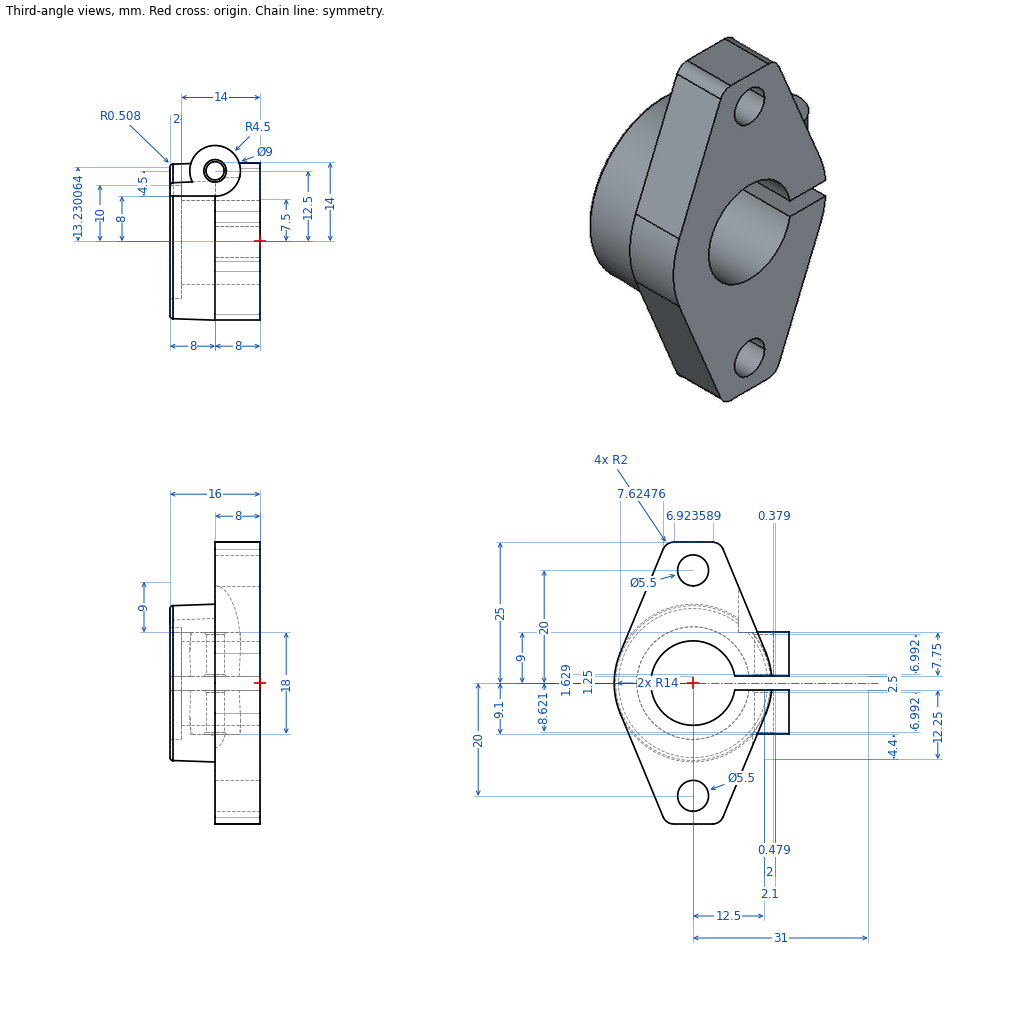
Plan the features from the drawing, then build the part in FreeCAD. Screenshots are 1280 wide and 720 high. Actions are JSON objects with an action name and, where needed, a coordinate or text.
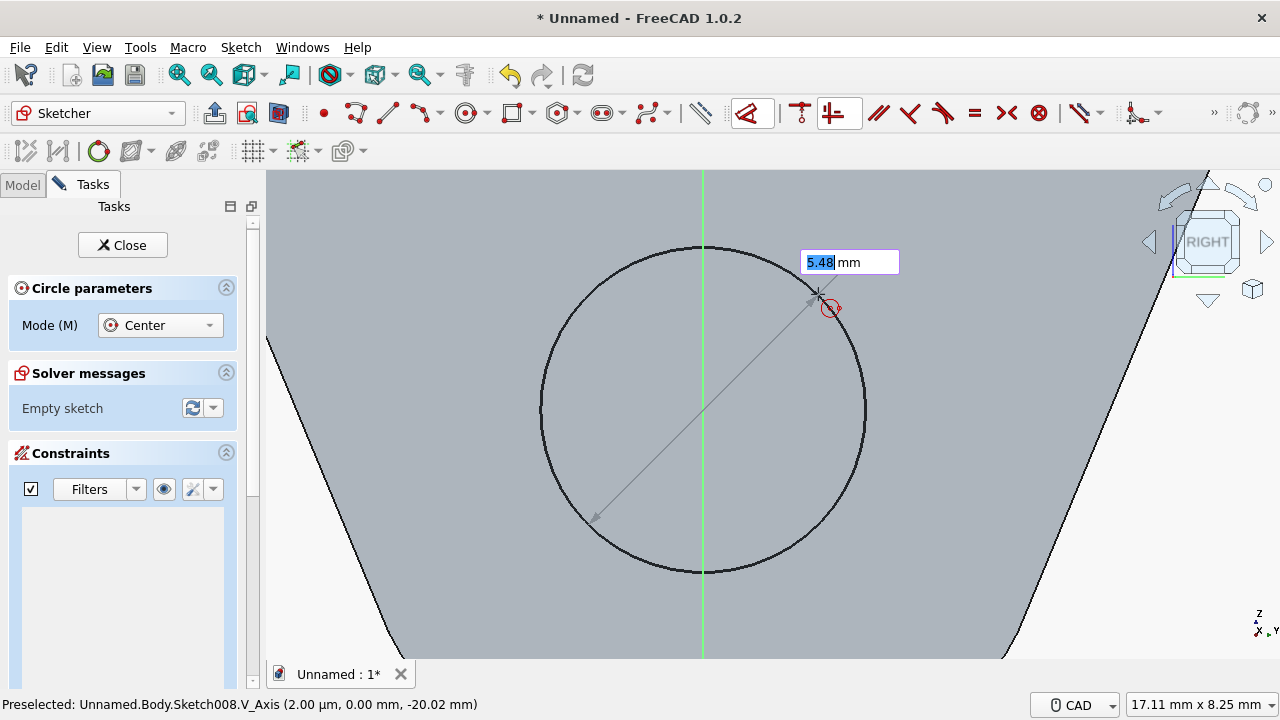
{"action": "type", "text": "5.5"}
{"action": "key", "text": "Return"}
{"action": "key", "text": "Escape"}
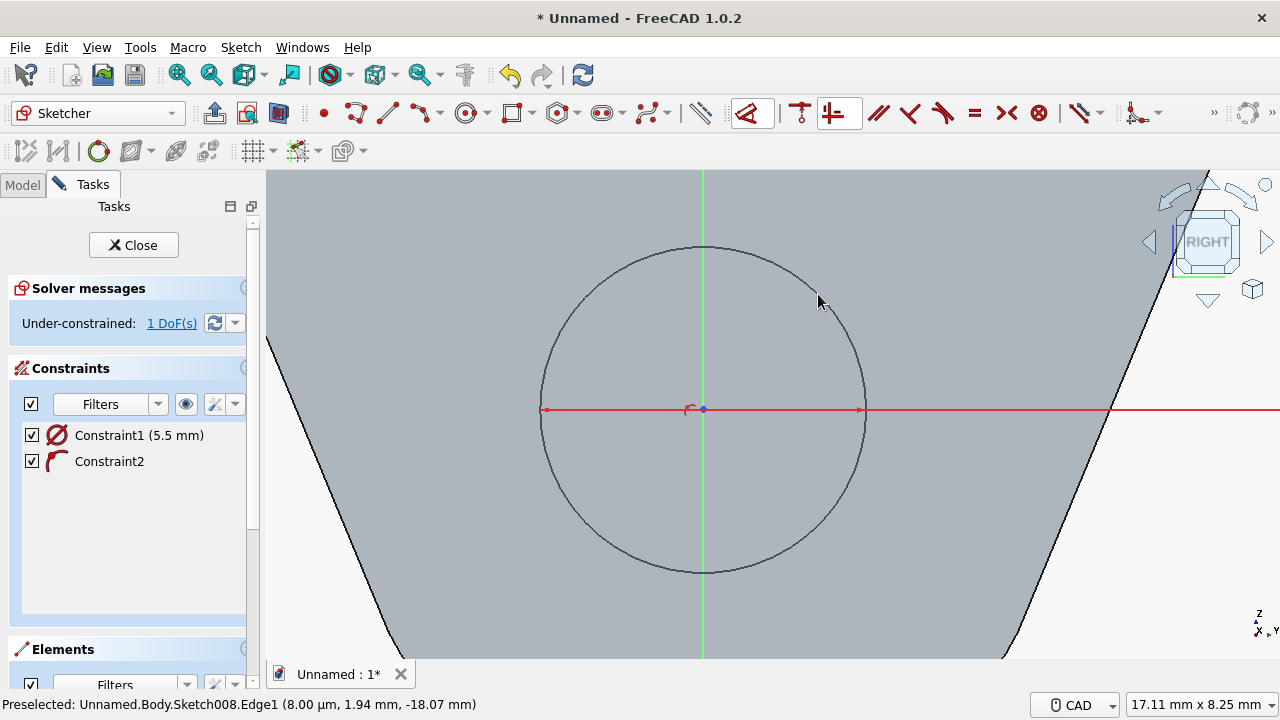
{"action": "left_click", "coordinate": [703, 410]}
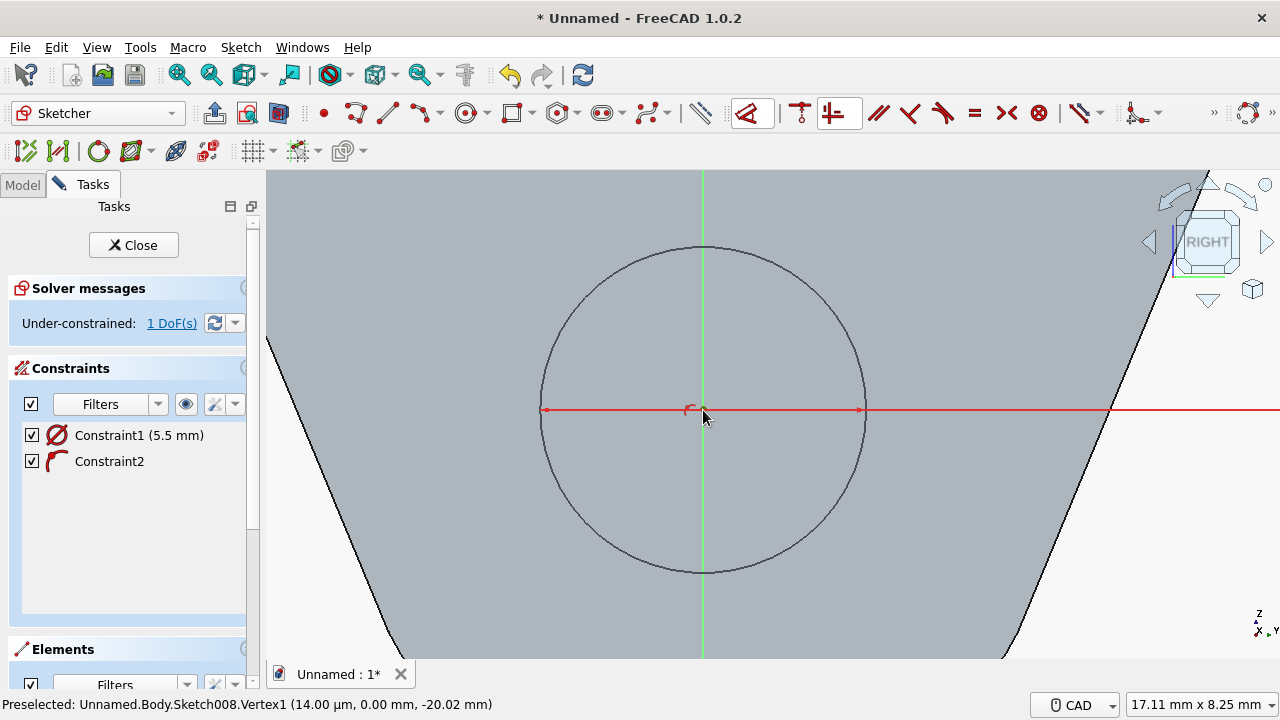
{"action": "left_click", "coordinate": [768, 114]}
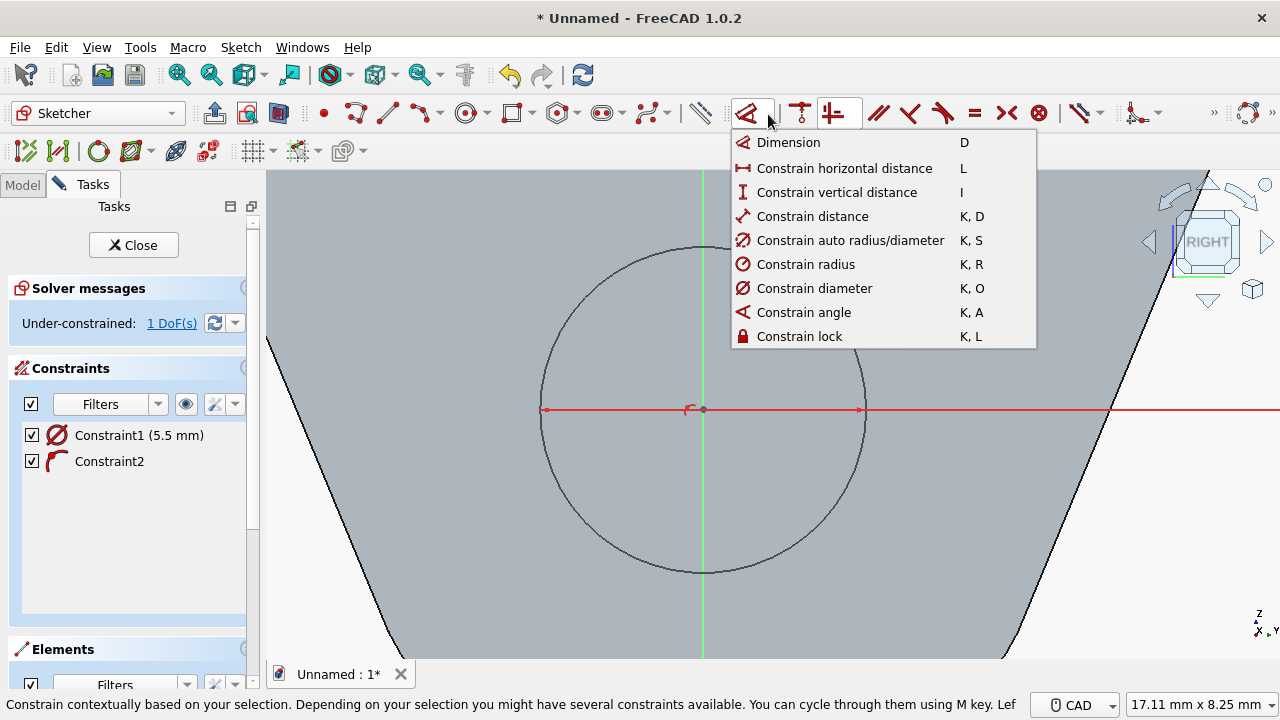
{"action": "left_click", "coordinate": [884, 192]}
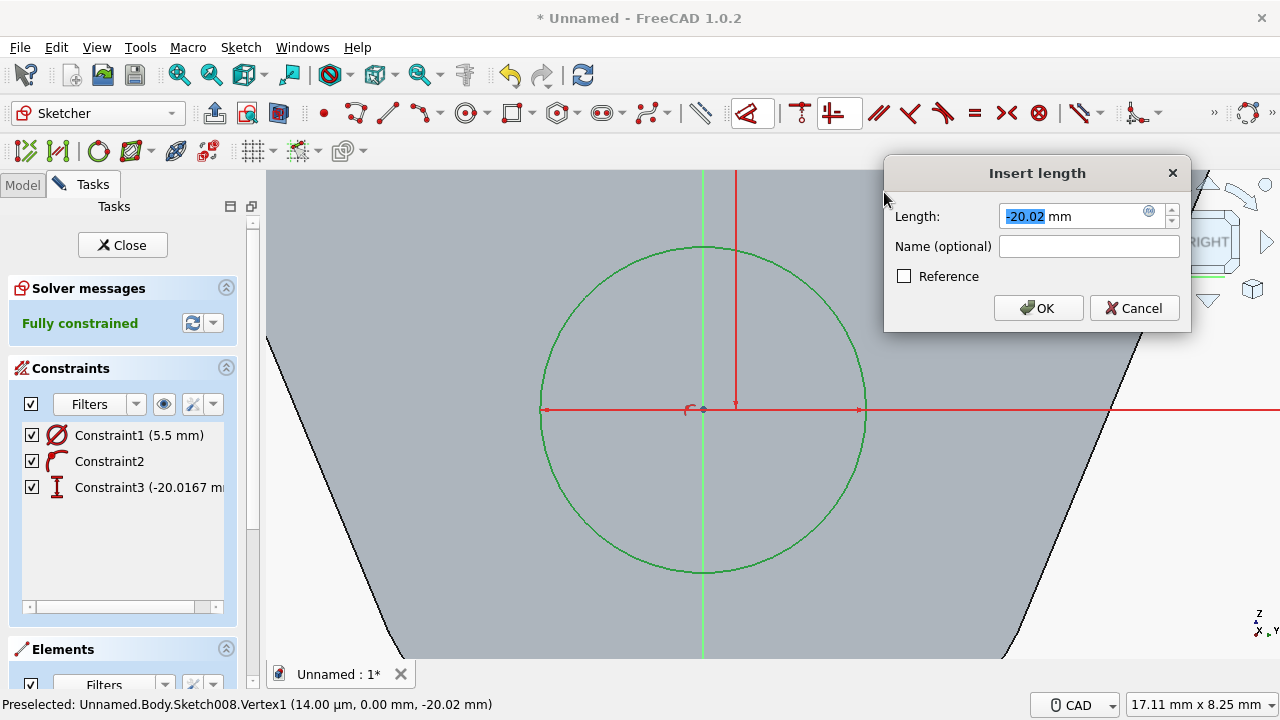
{"action": "type", "text": "-20"}
{"action": "key", "text": "Return"}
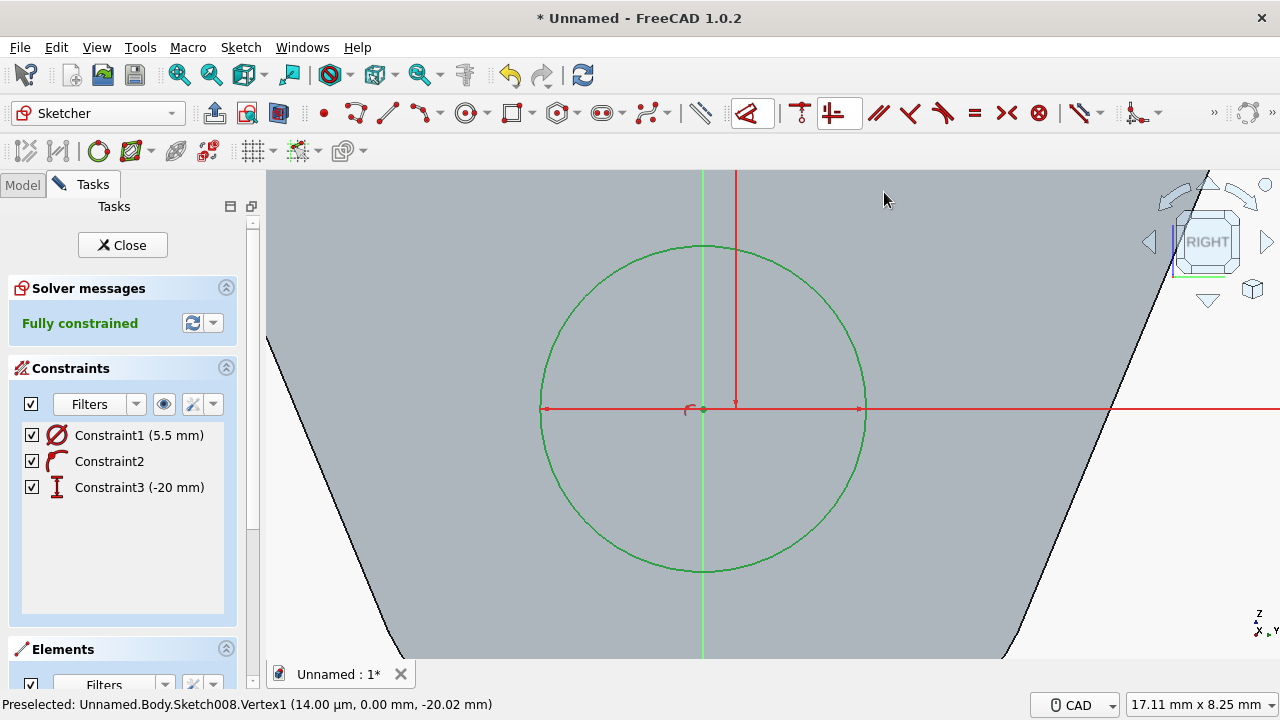
{"action": "left_click", "coordinate": [123, 245]}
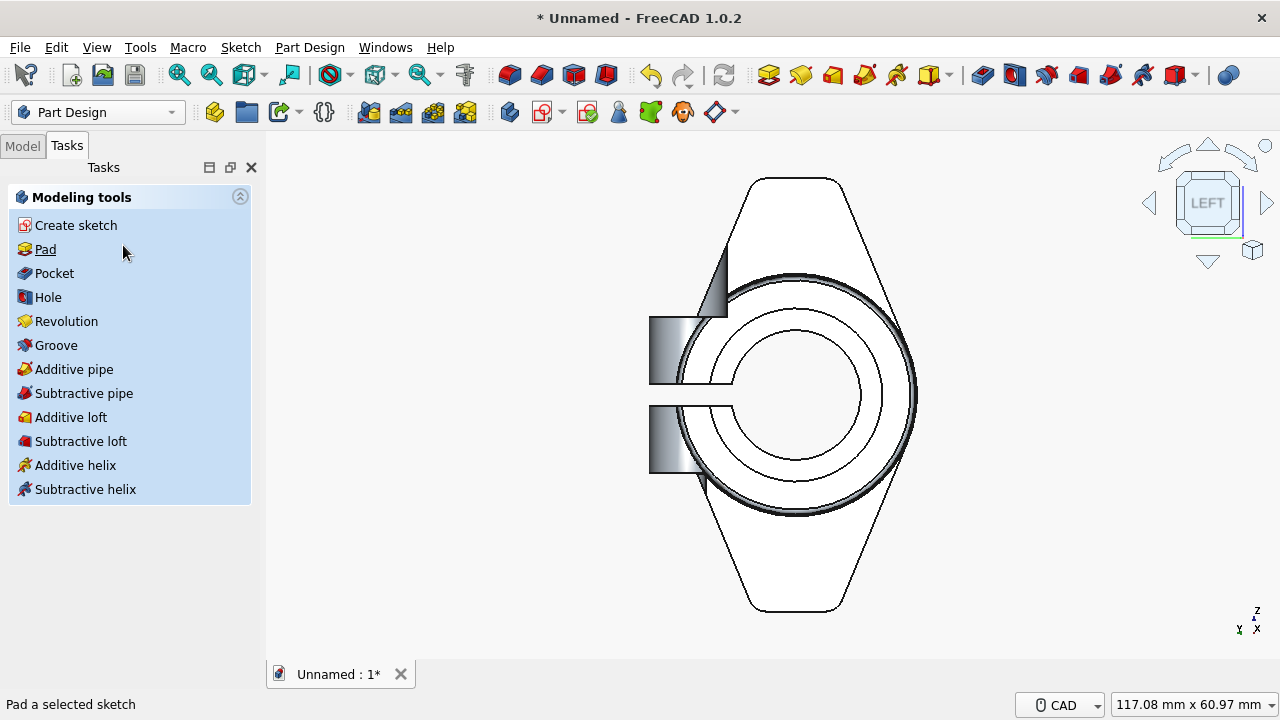
{"action": "left_click", "coordinate": [984, 76]}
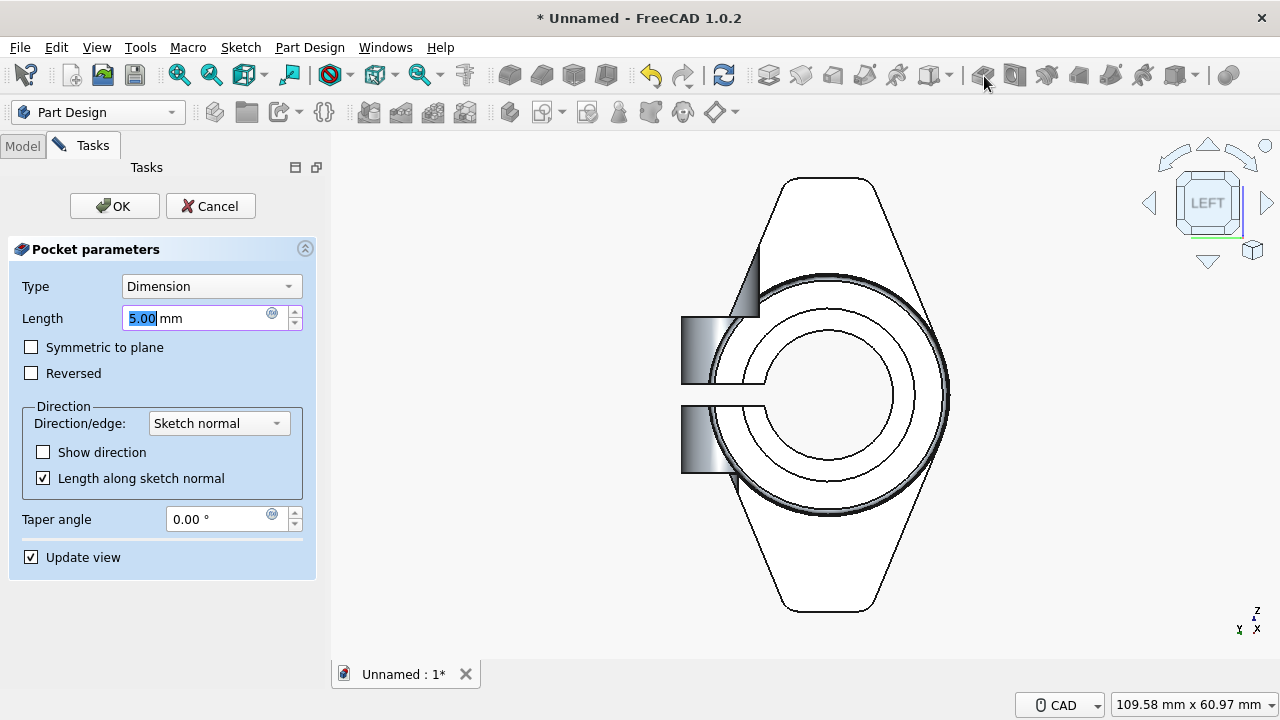
{"action": "type", "text": "8"}
{"action": "key", "text": "Tab"}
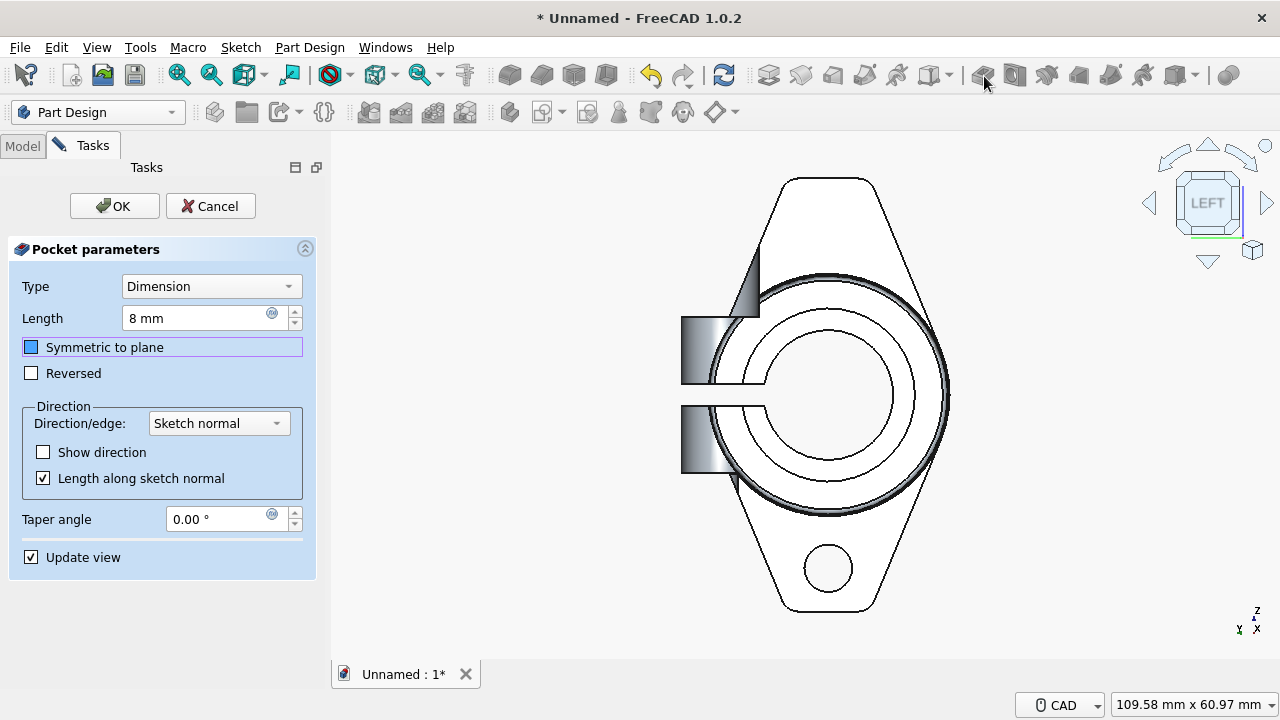
{"action": "left_click", "coordinate": [115, 206]}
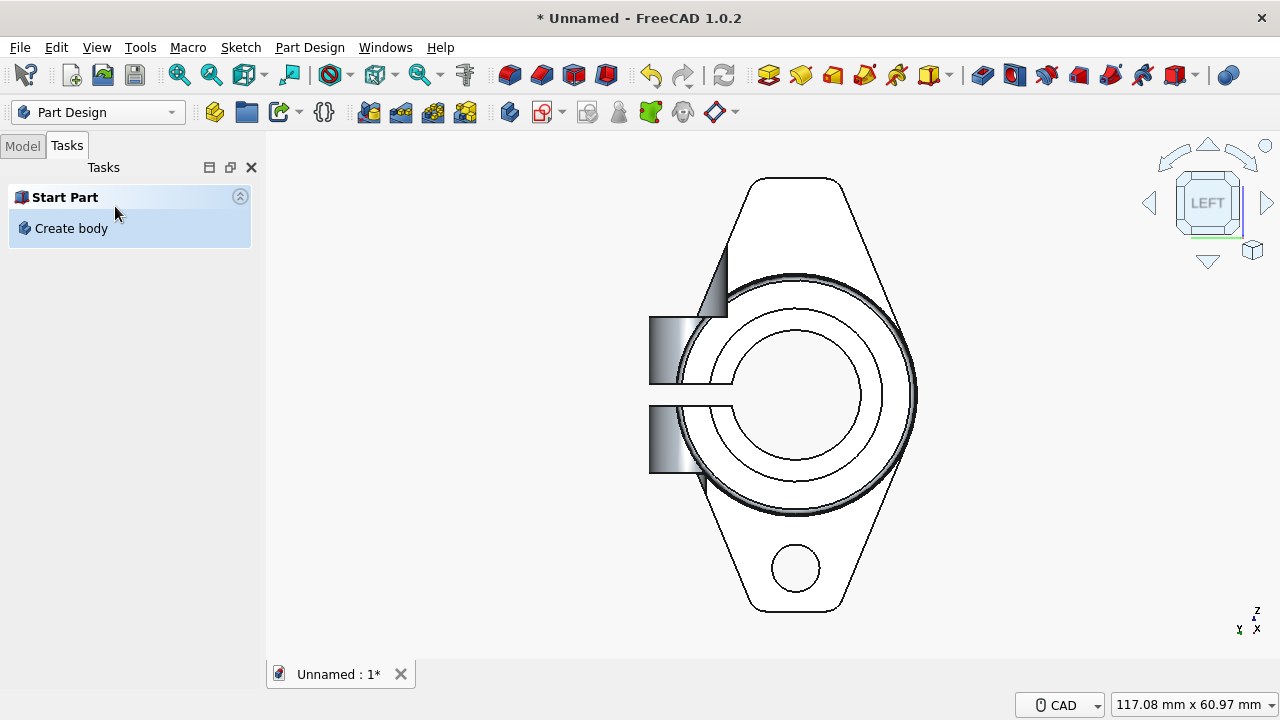
{"action": "left_click", "coordinate": [542, 112]}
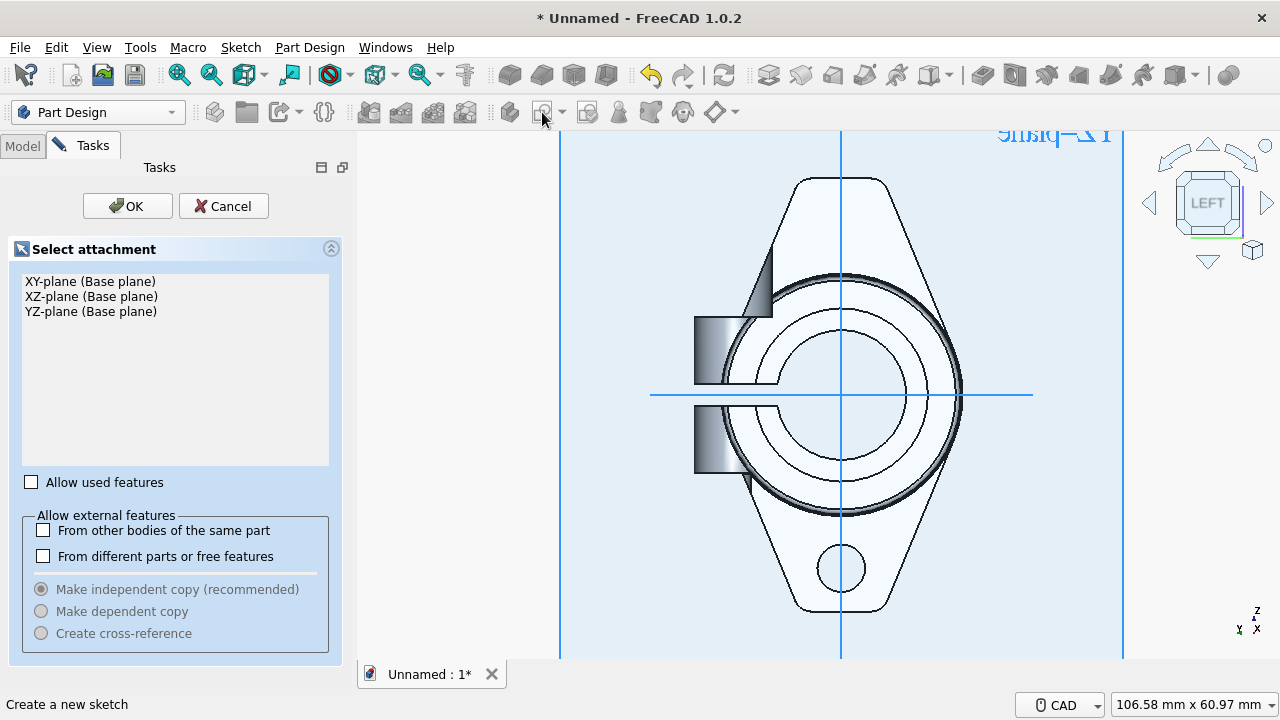
{"action": "left_click", "coordinate": [82, 312]}